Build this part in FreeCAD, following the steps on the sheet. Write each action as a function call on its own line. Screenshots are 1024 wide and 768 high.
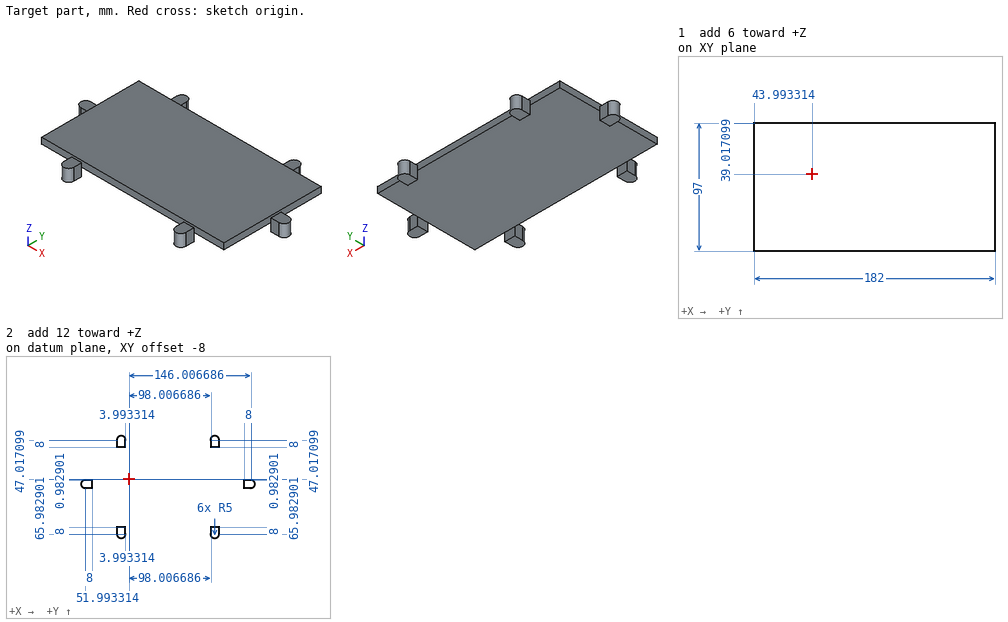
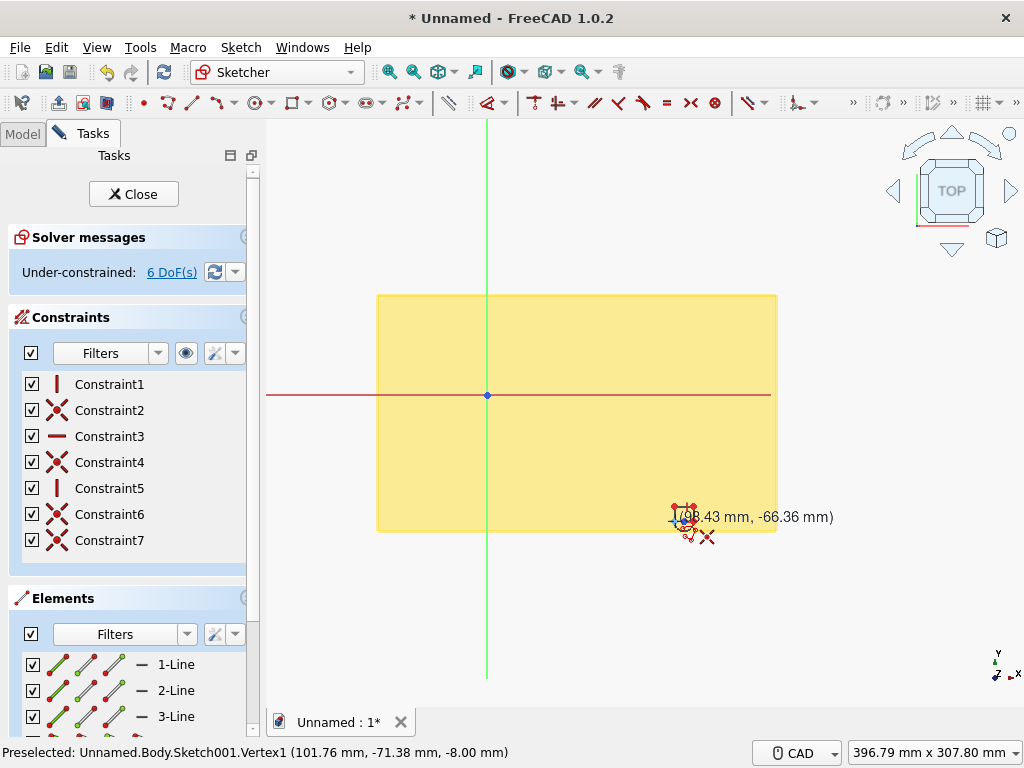
scroll(766, 397, up, 11)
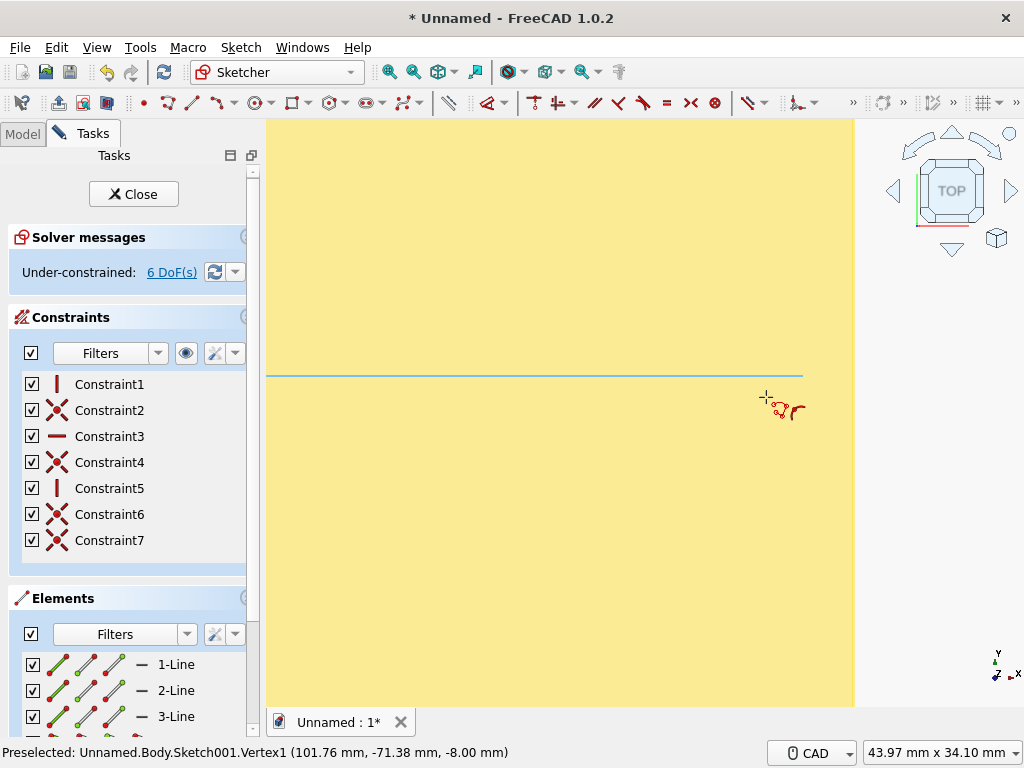
click(762, 393)
click(624, 393)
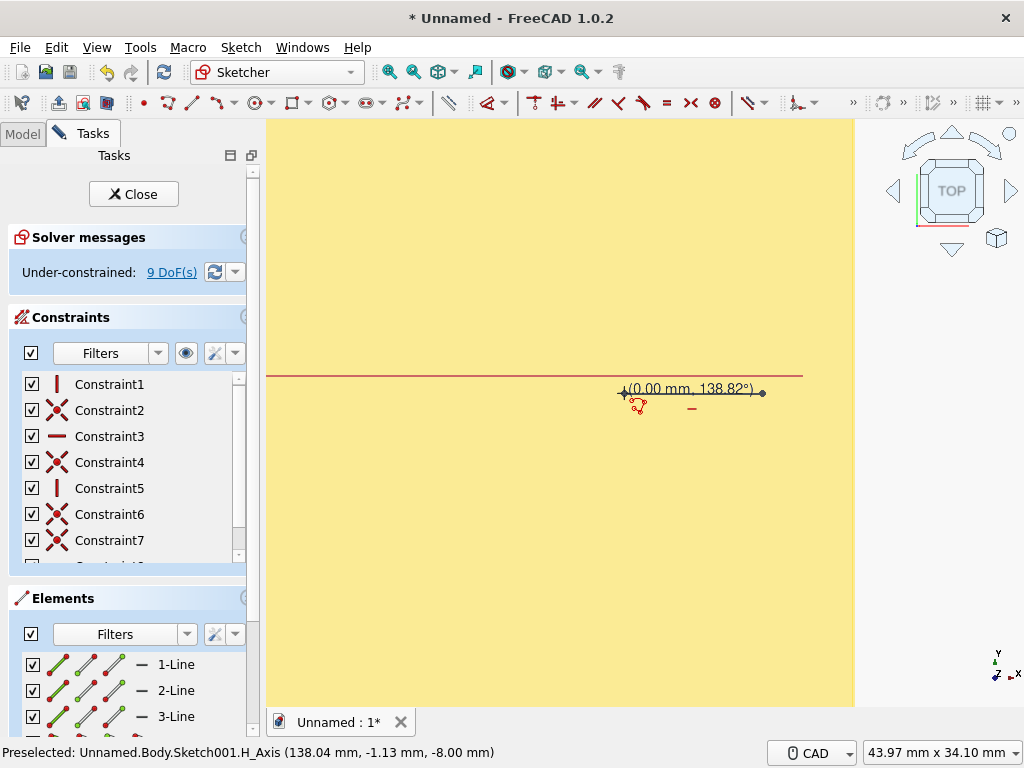
scroll(766, 397, down, 11)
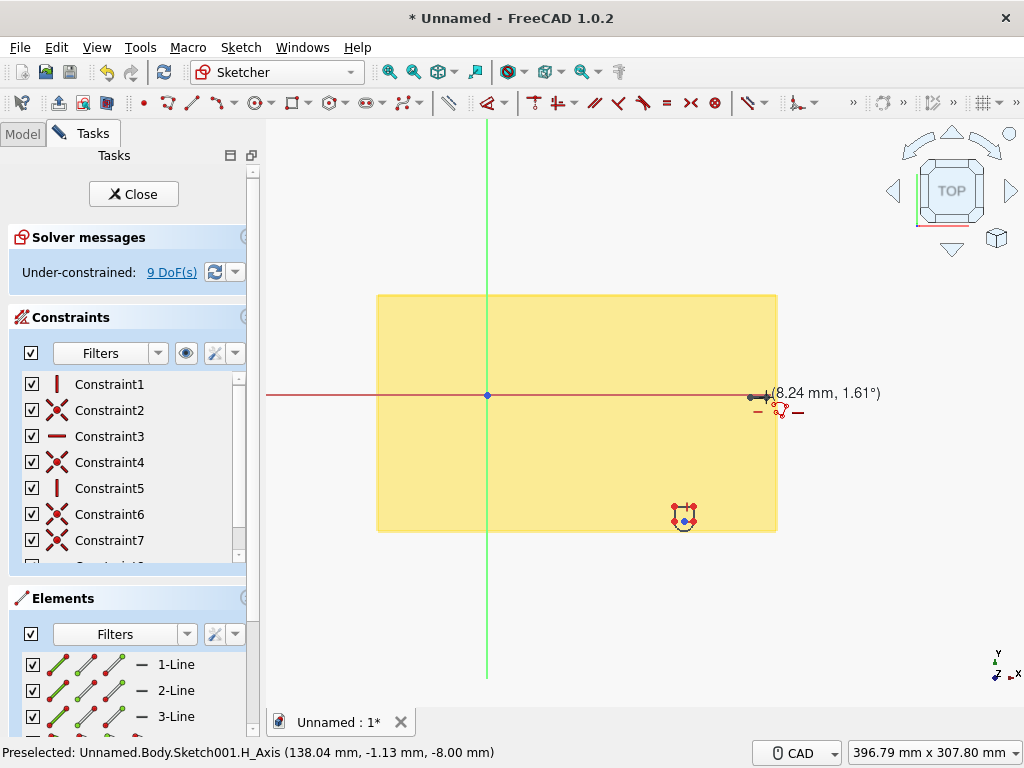
click(751, 416)
click(766, 416)
right_click(766, 416)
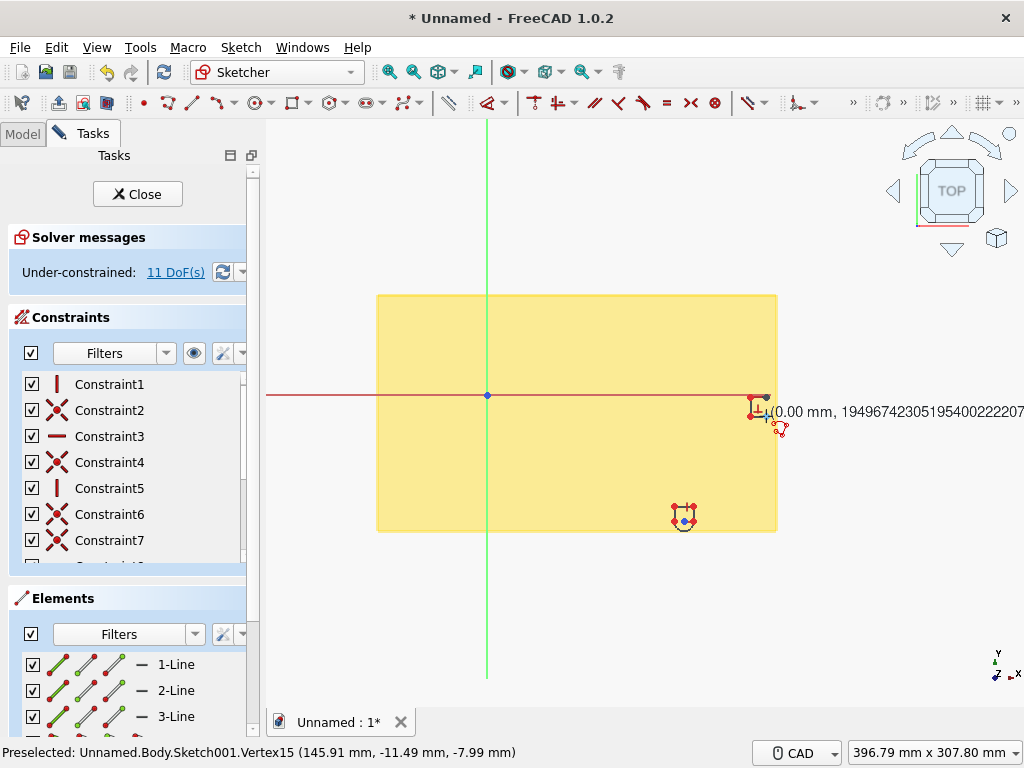
click(218, 104)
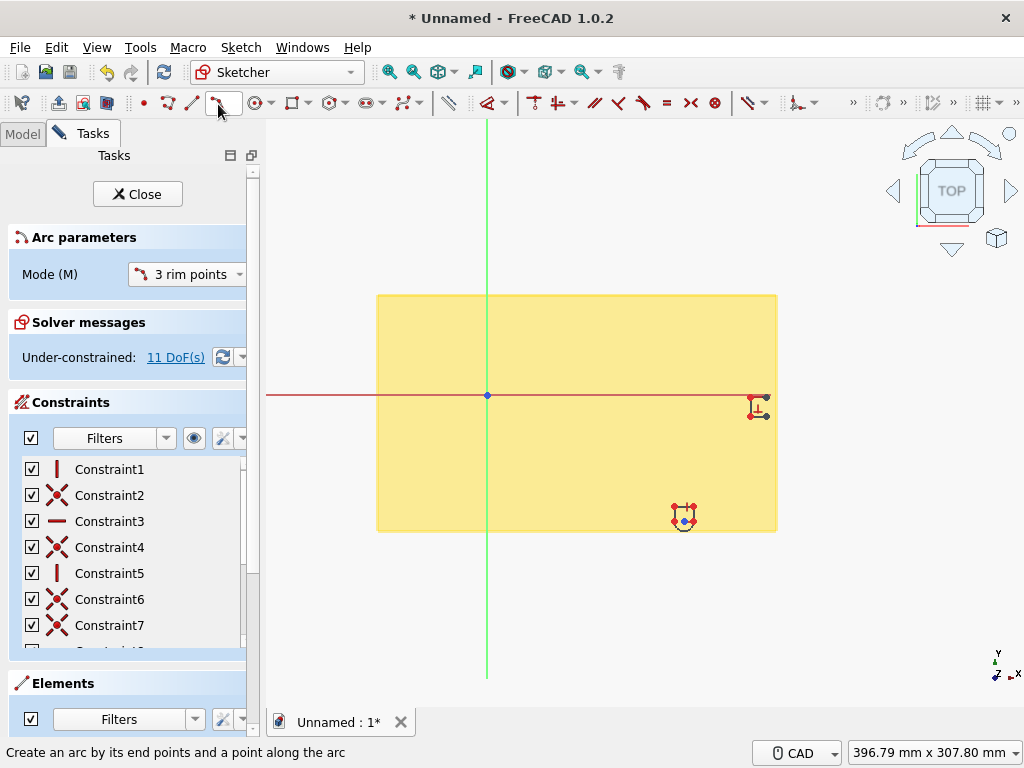
scroll(766, 416, up, 4)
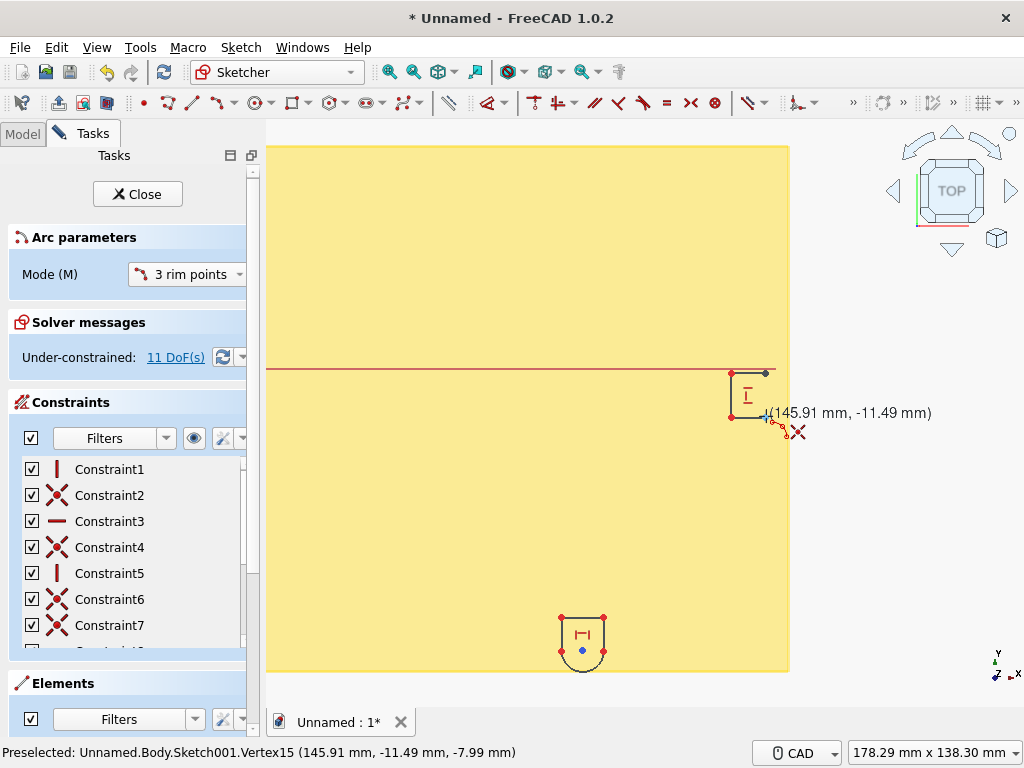
click(765, 418)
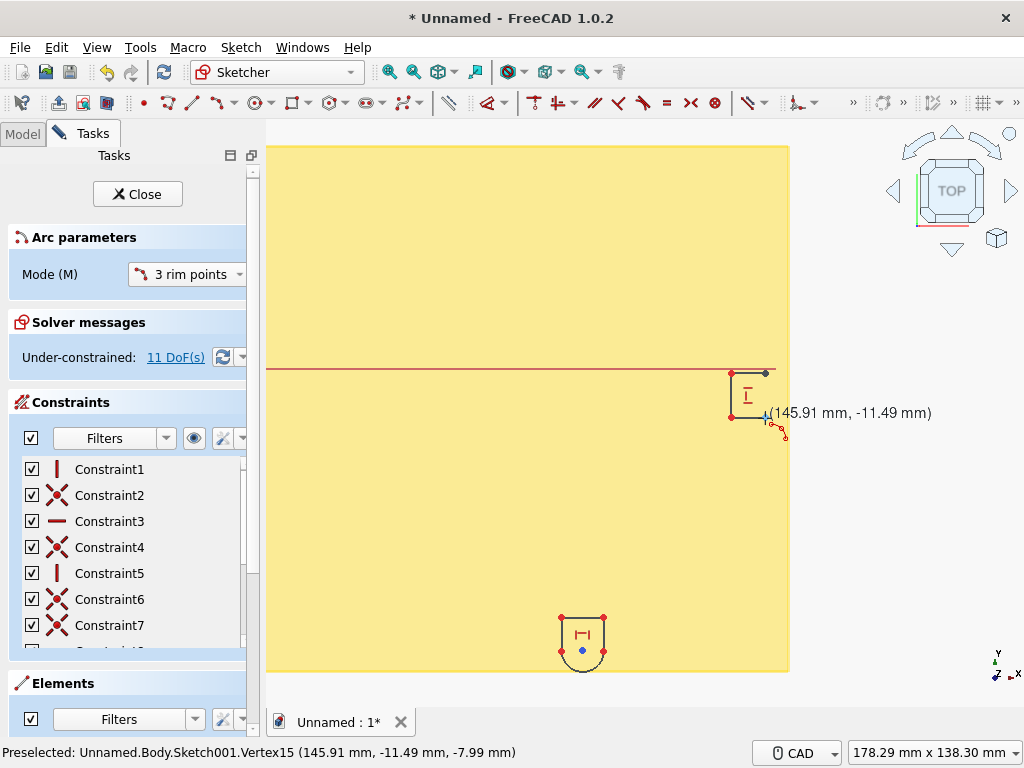
scroll(766, 373, up, 7)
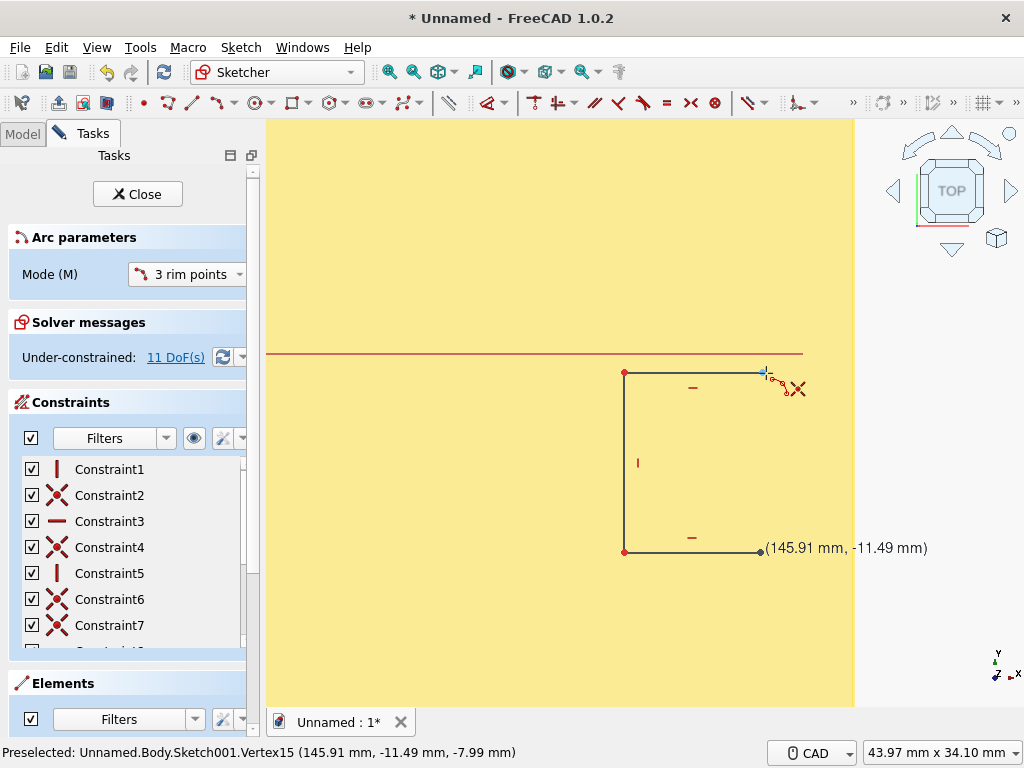
click(762, 373)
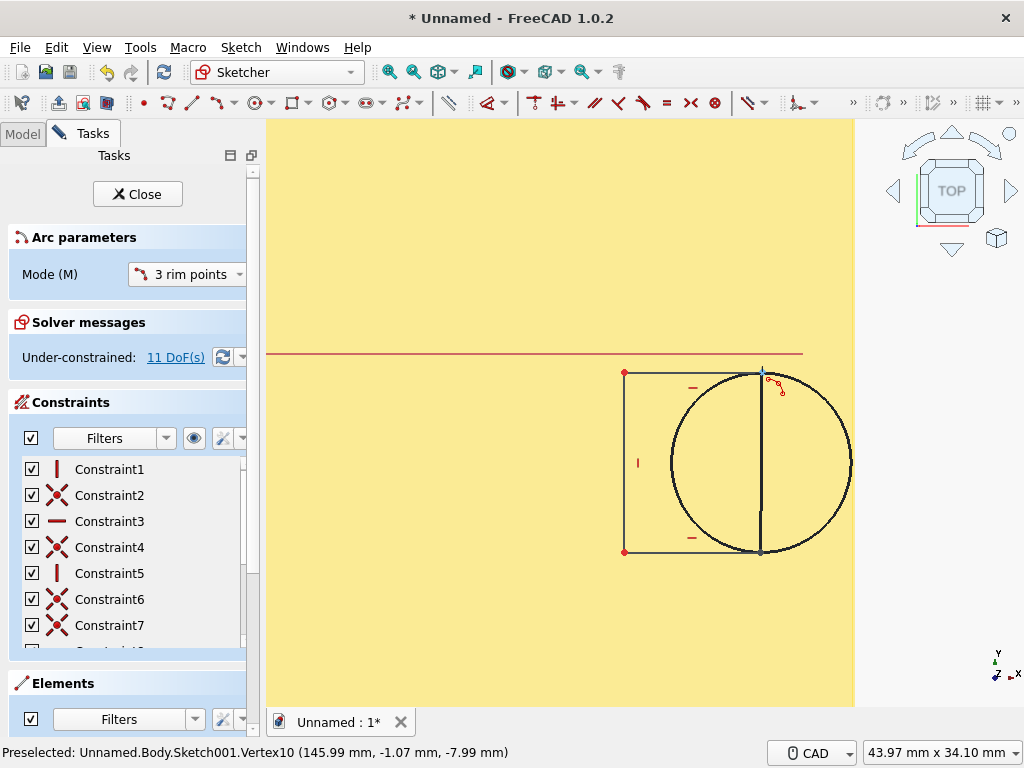
scroll(766, 400, down, 11)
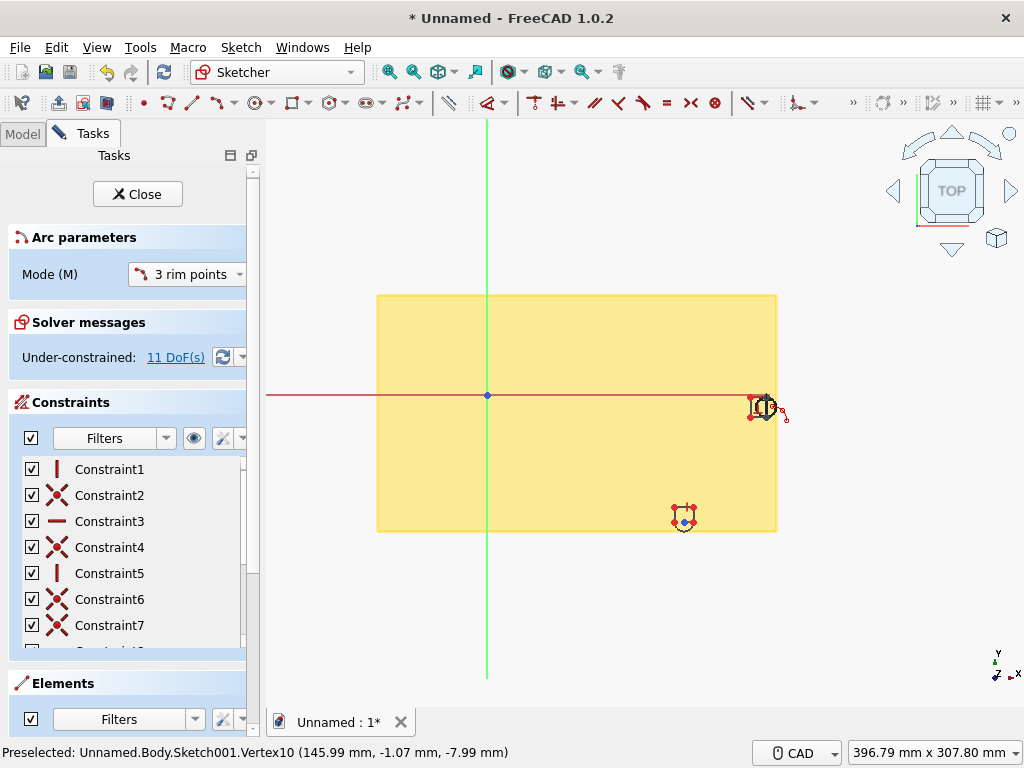
scroll(776, 407, up, 3)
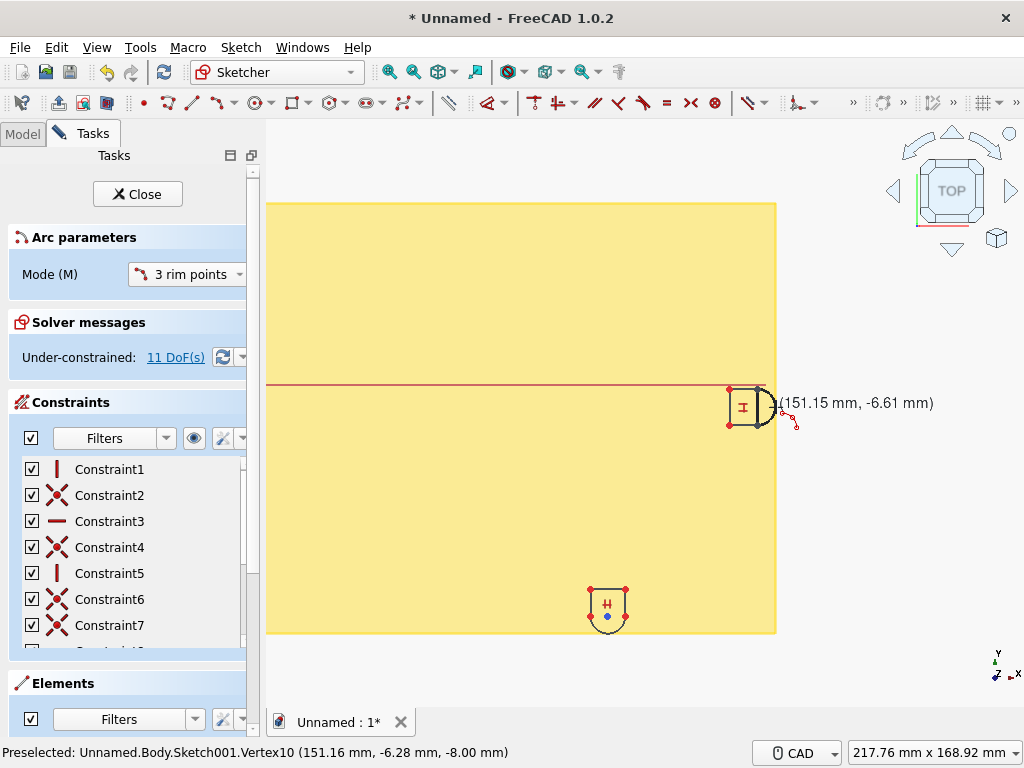
click(775, 406)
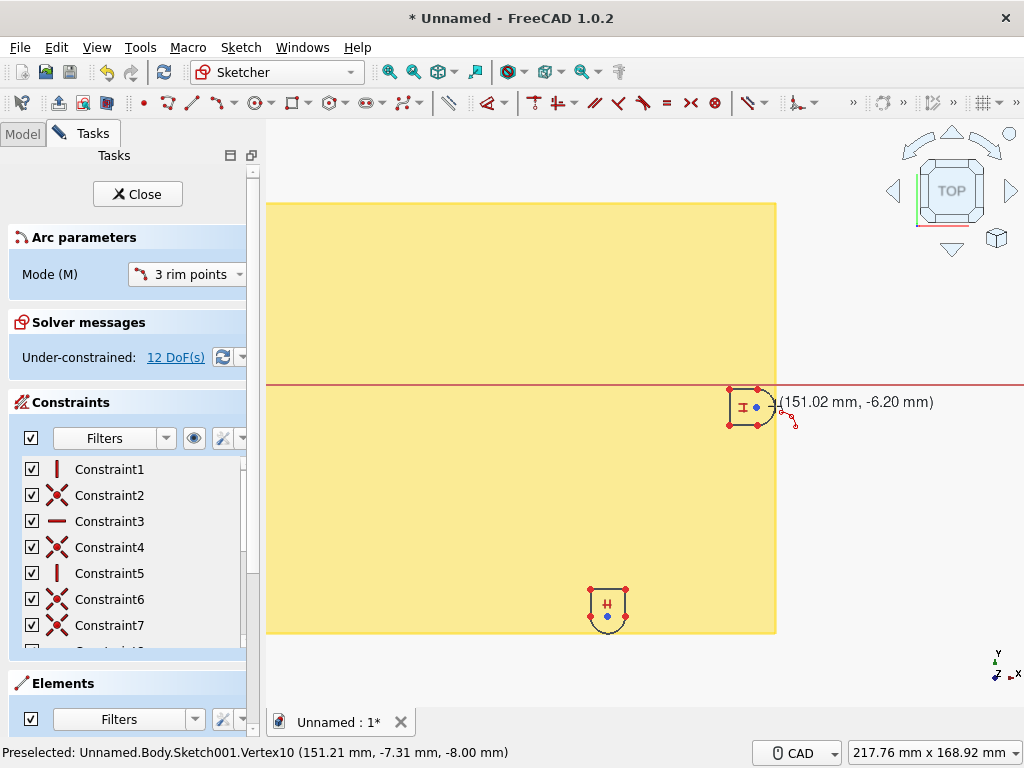
click(168, 104)